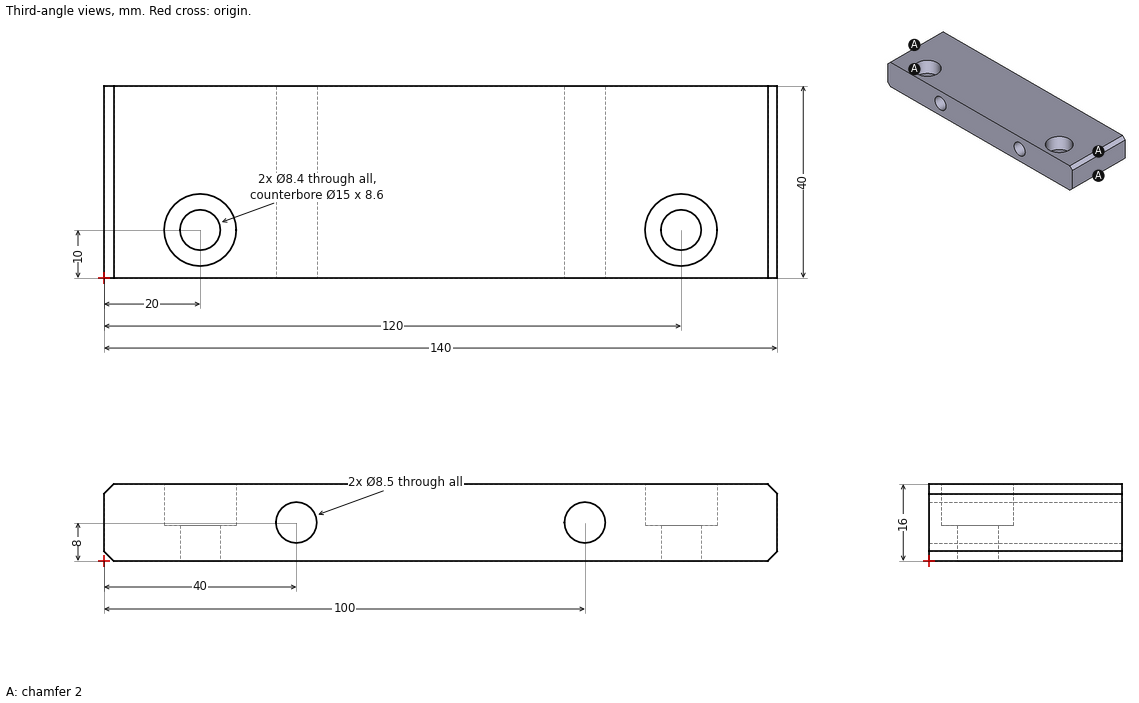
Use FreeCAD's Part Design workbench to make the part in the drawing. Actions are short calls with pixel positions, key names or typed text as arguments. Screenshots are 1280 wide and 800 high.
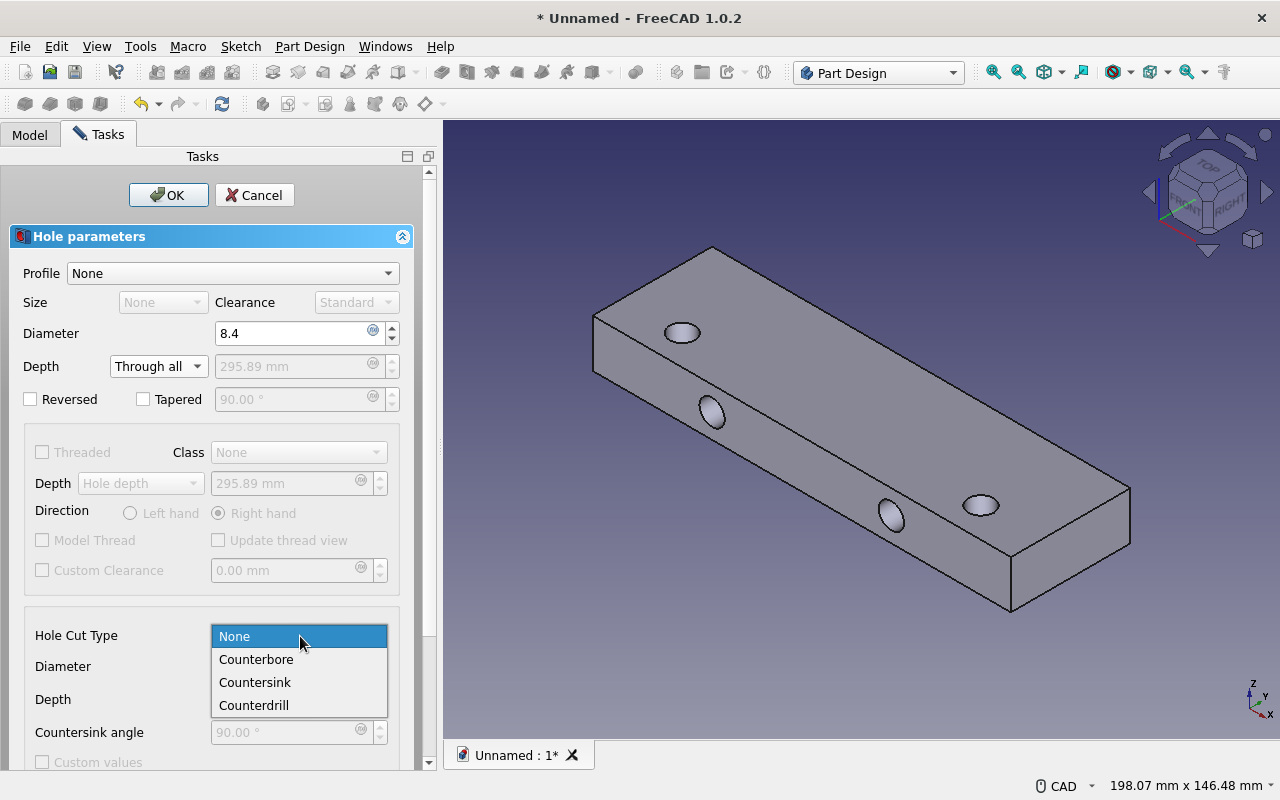
click(298, 660)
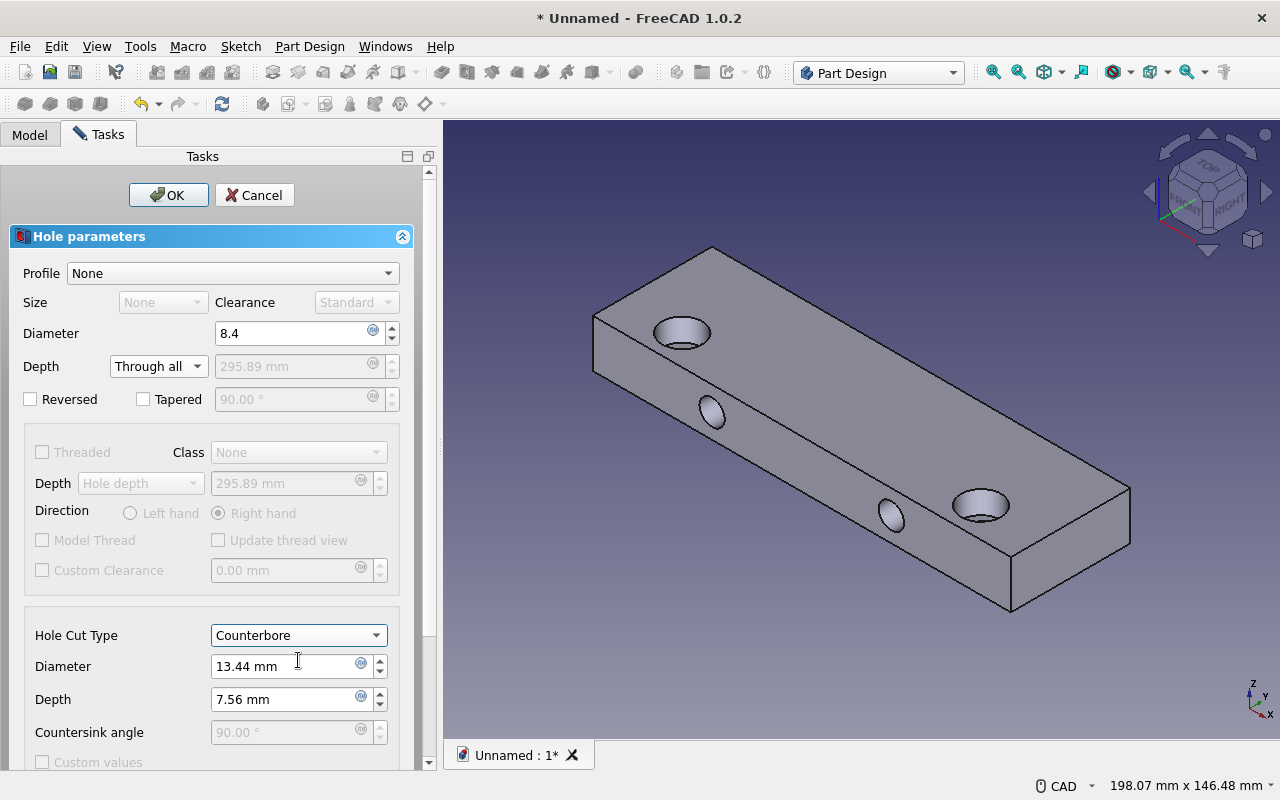
triple_click(292, 666)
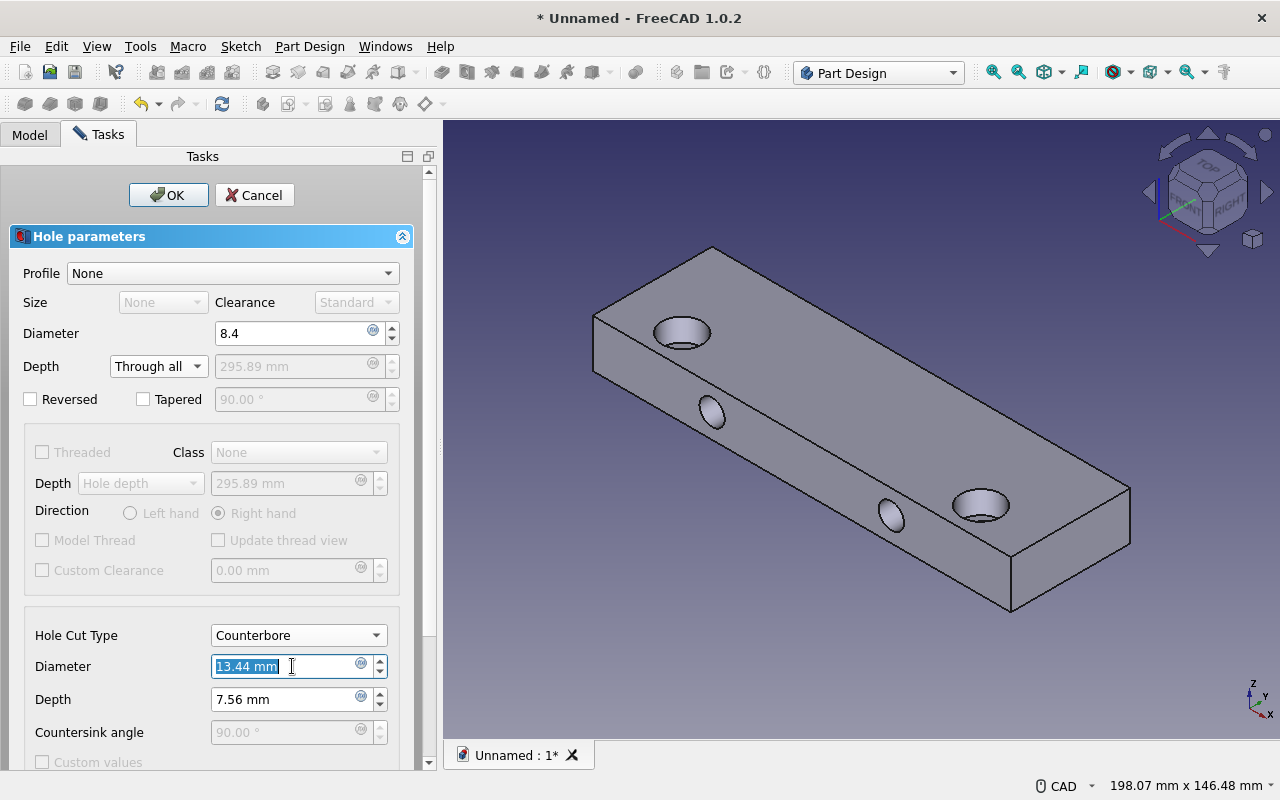
text(15)
key(Tab)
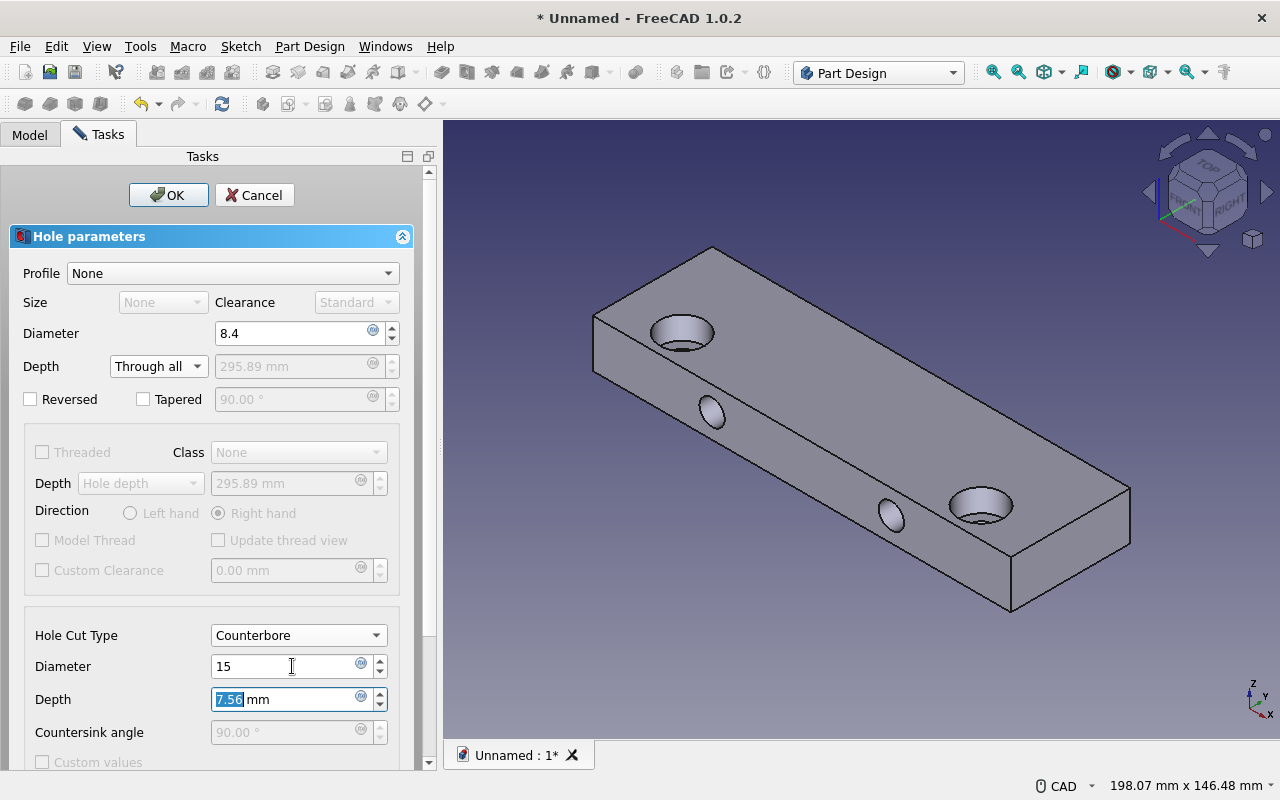
text(8.6)
key(Tab)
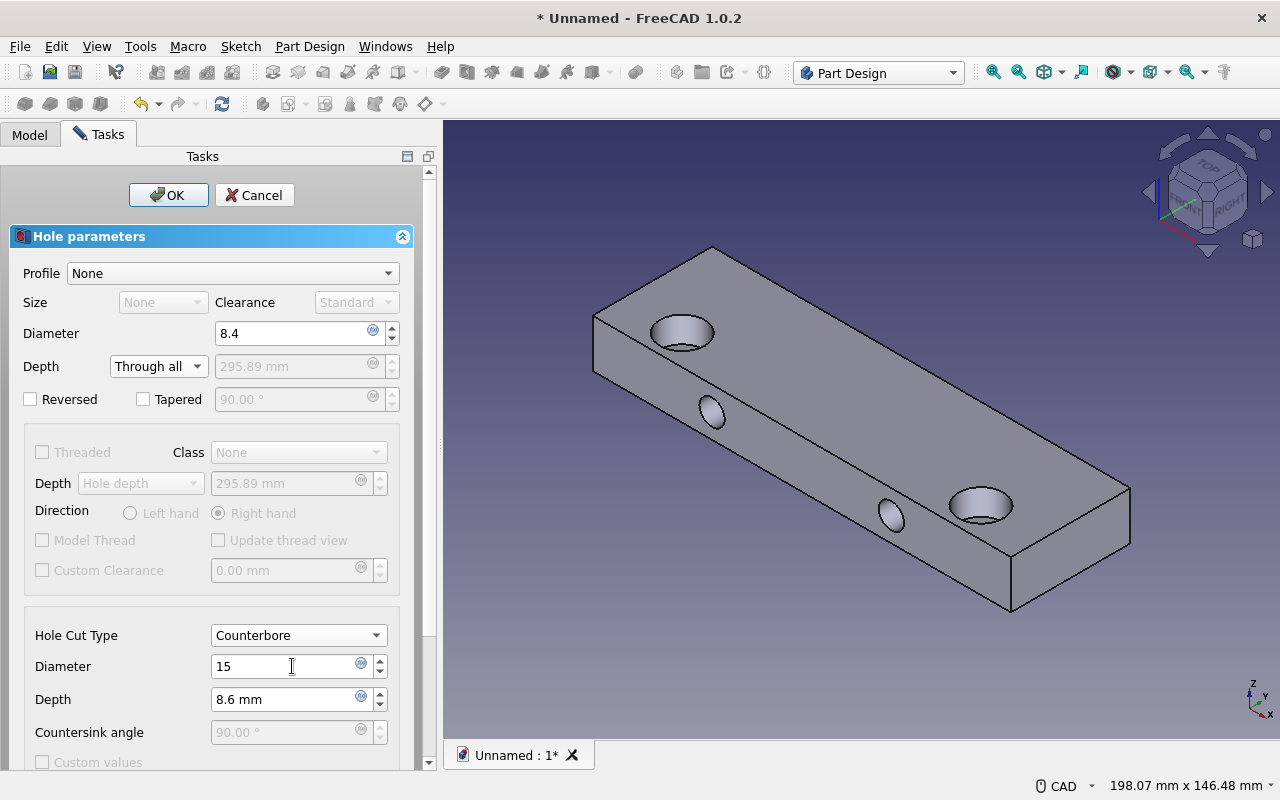
click(169, 195)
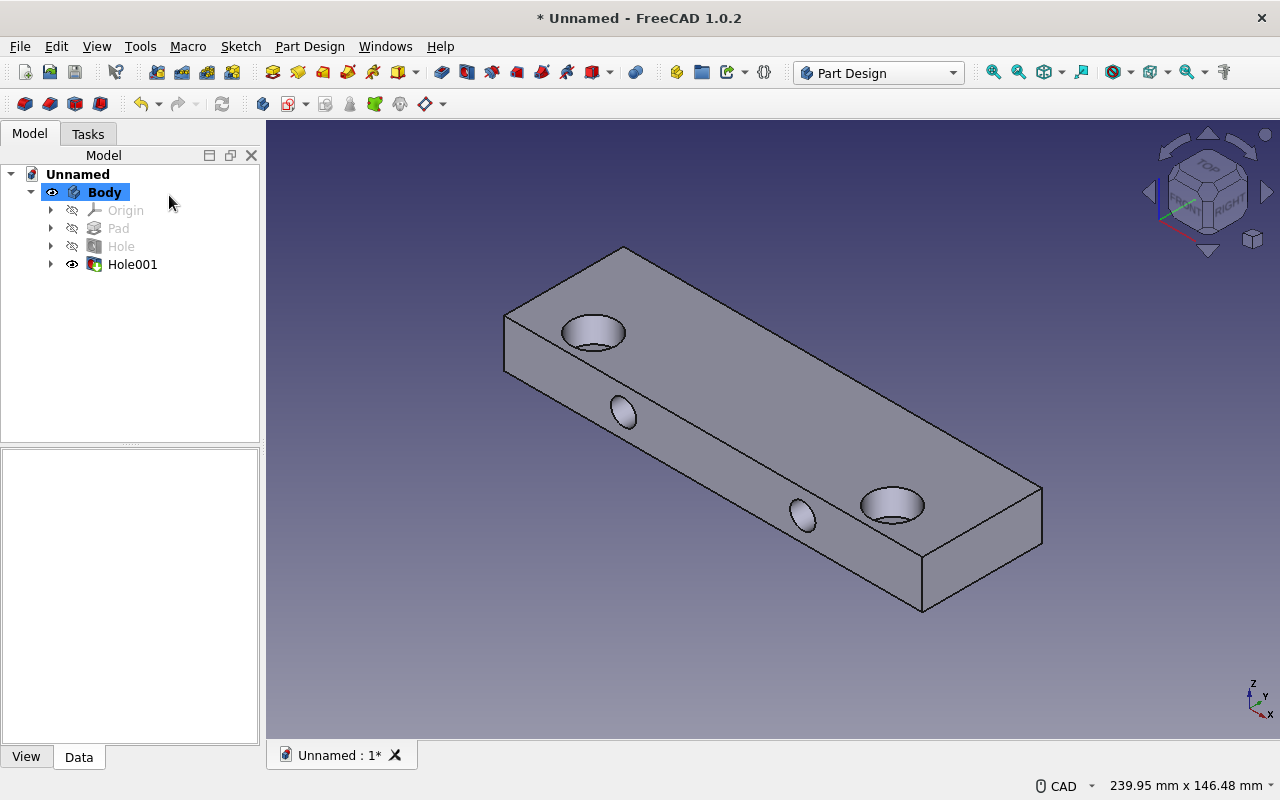
click(982, 522)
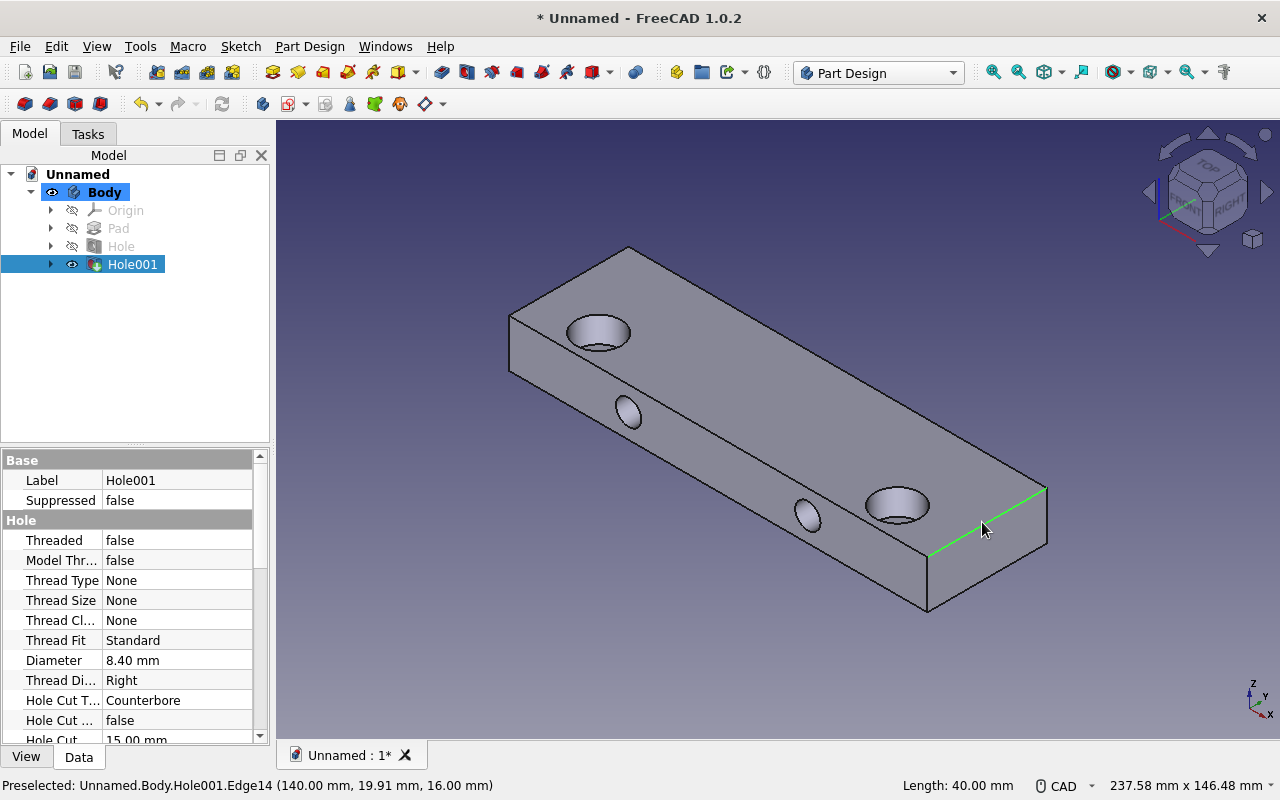
key(2)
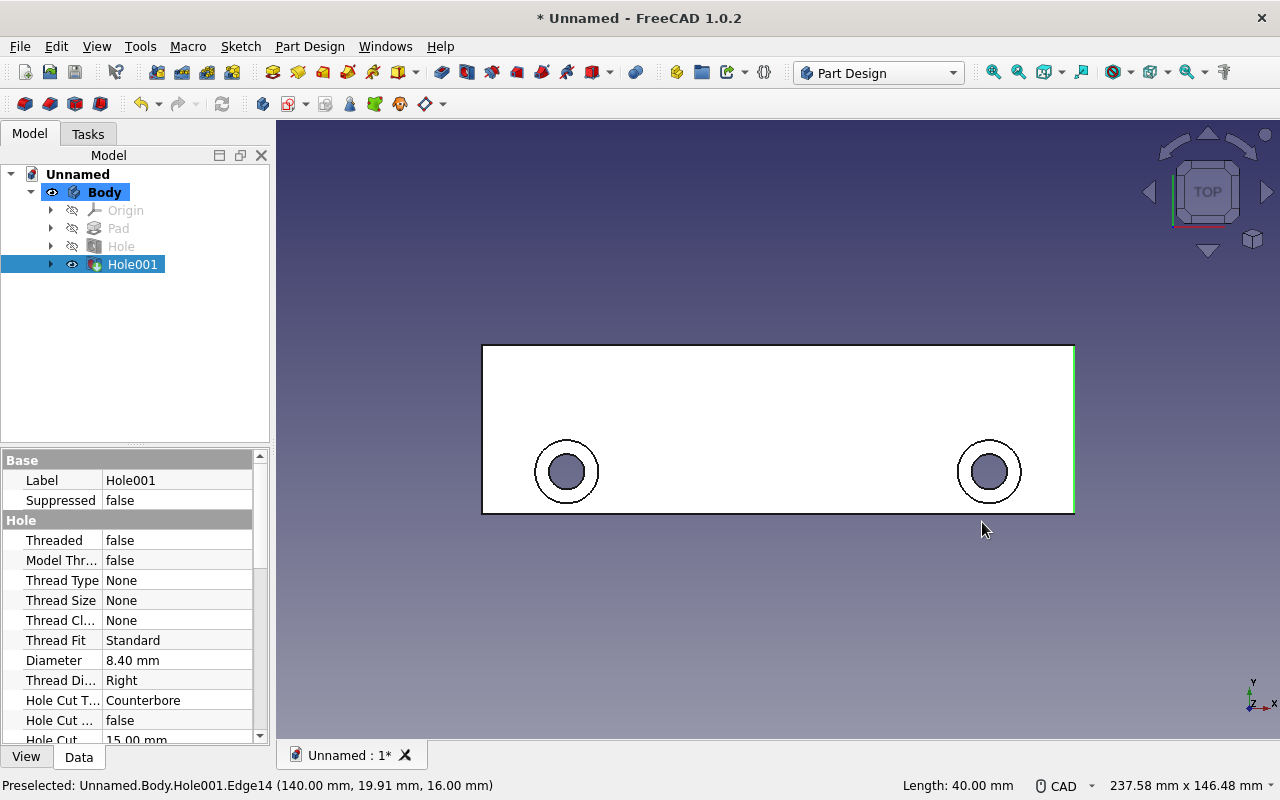
click(482, 428, ctrl)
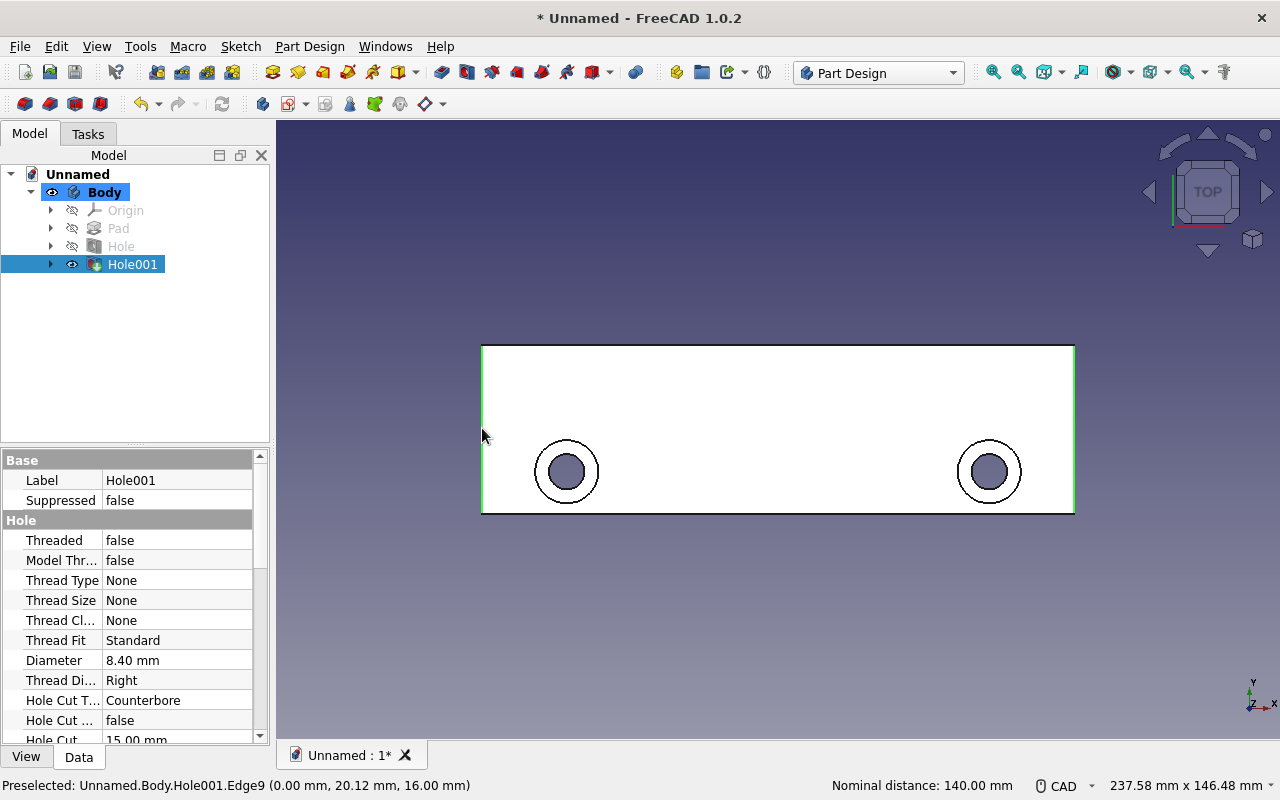
key(0)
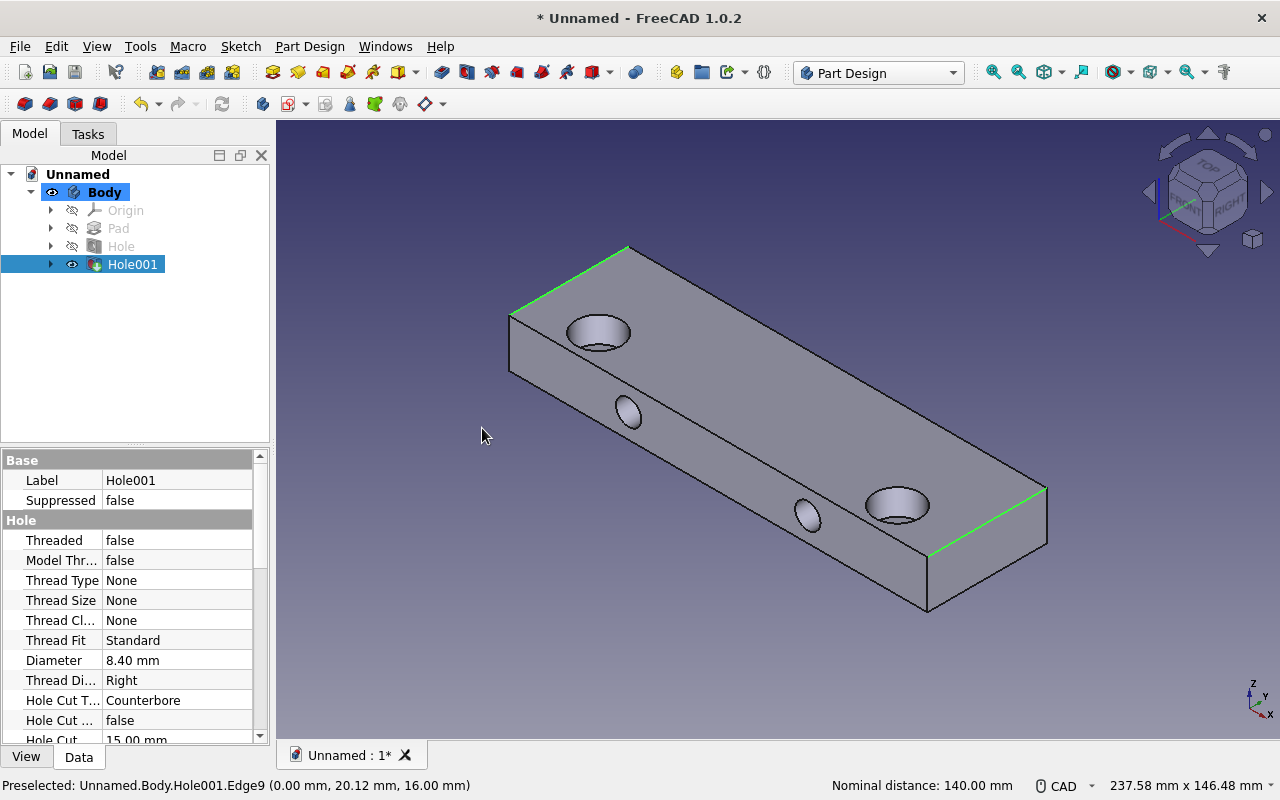
key(1)